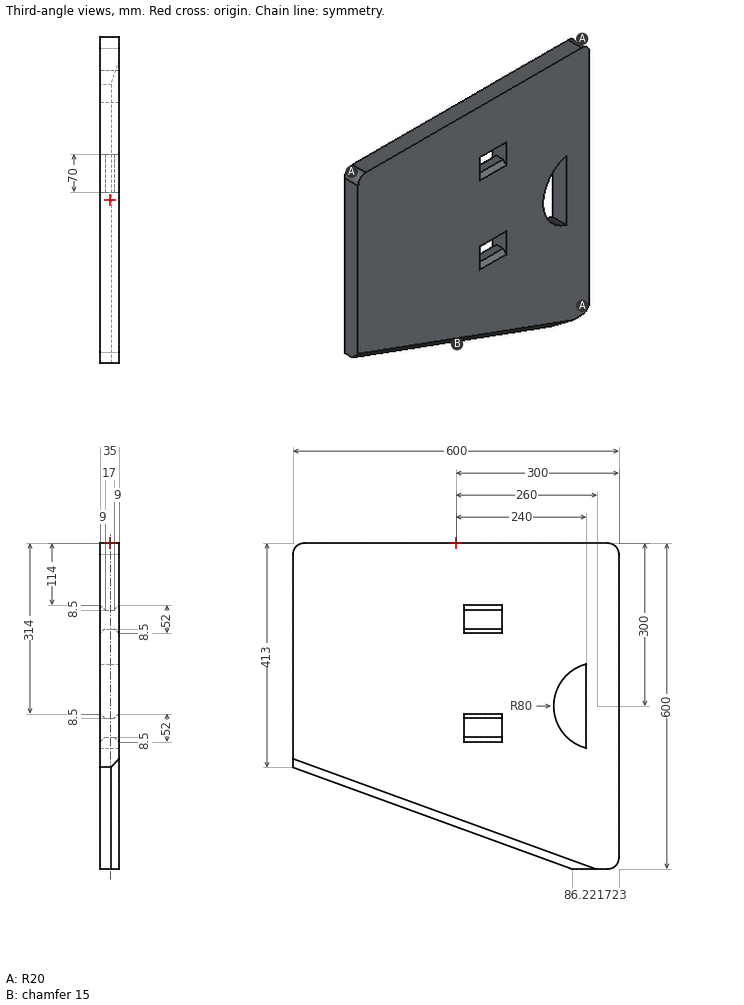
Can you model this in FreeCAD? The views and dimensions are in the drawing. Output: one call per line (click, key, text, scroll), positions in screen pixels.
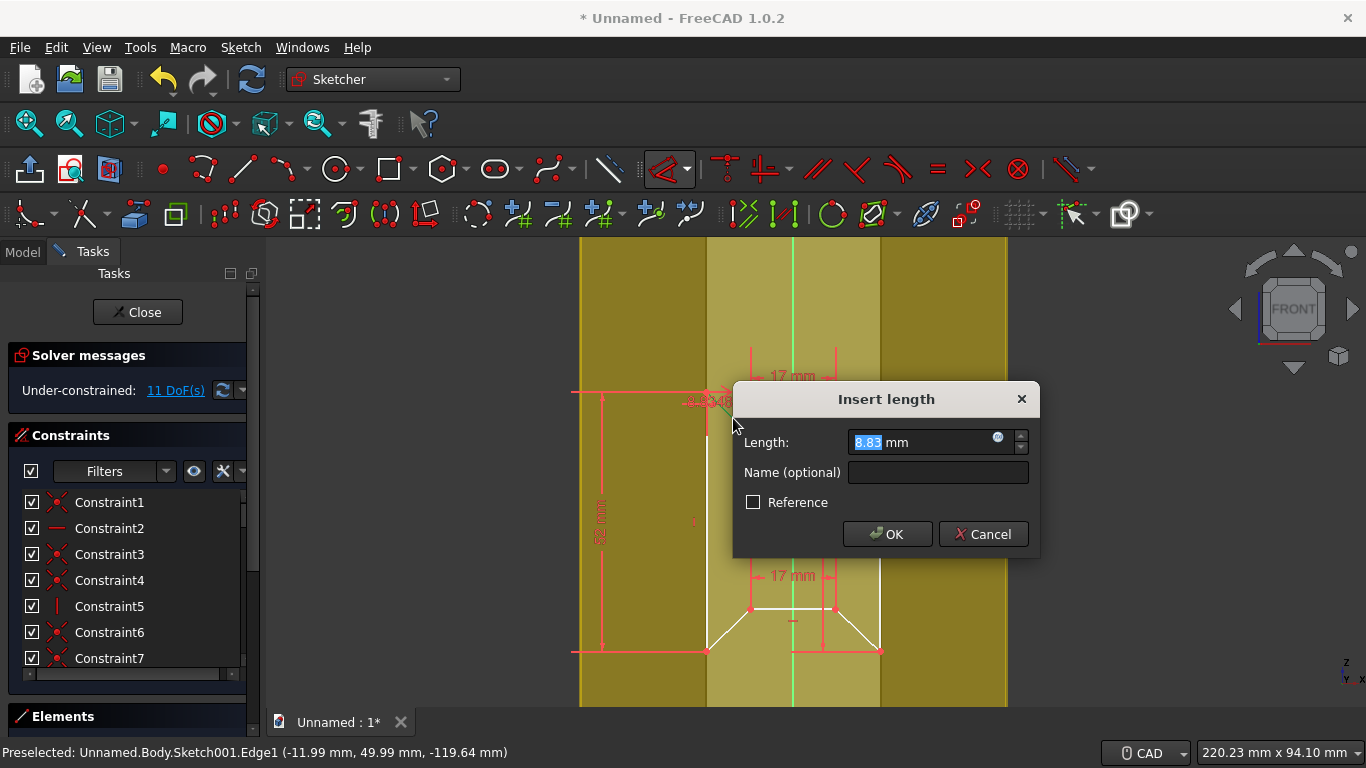
text(9)
key(Return)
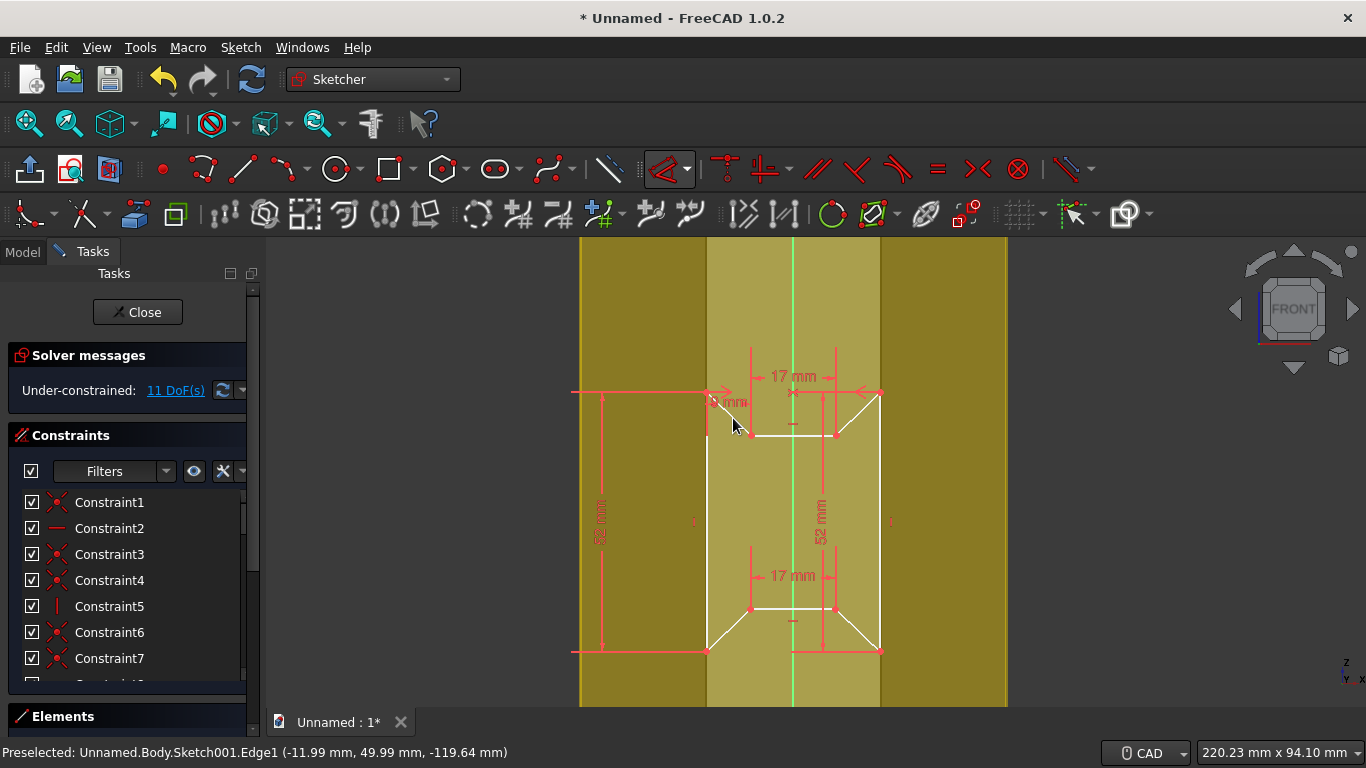
click(849, 422)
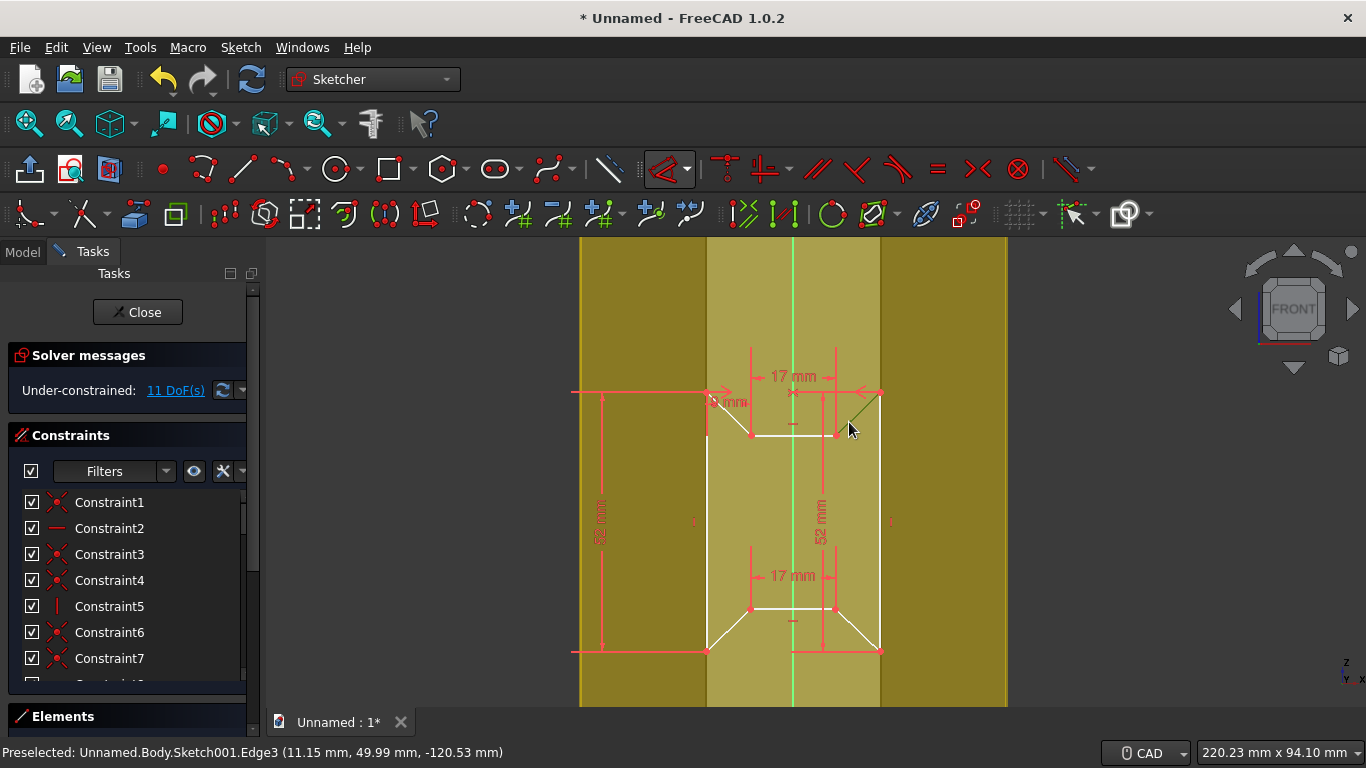
key(l)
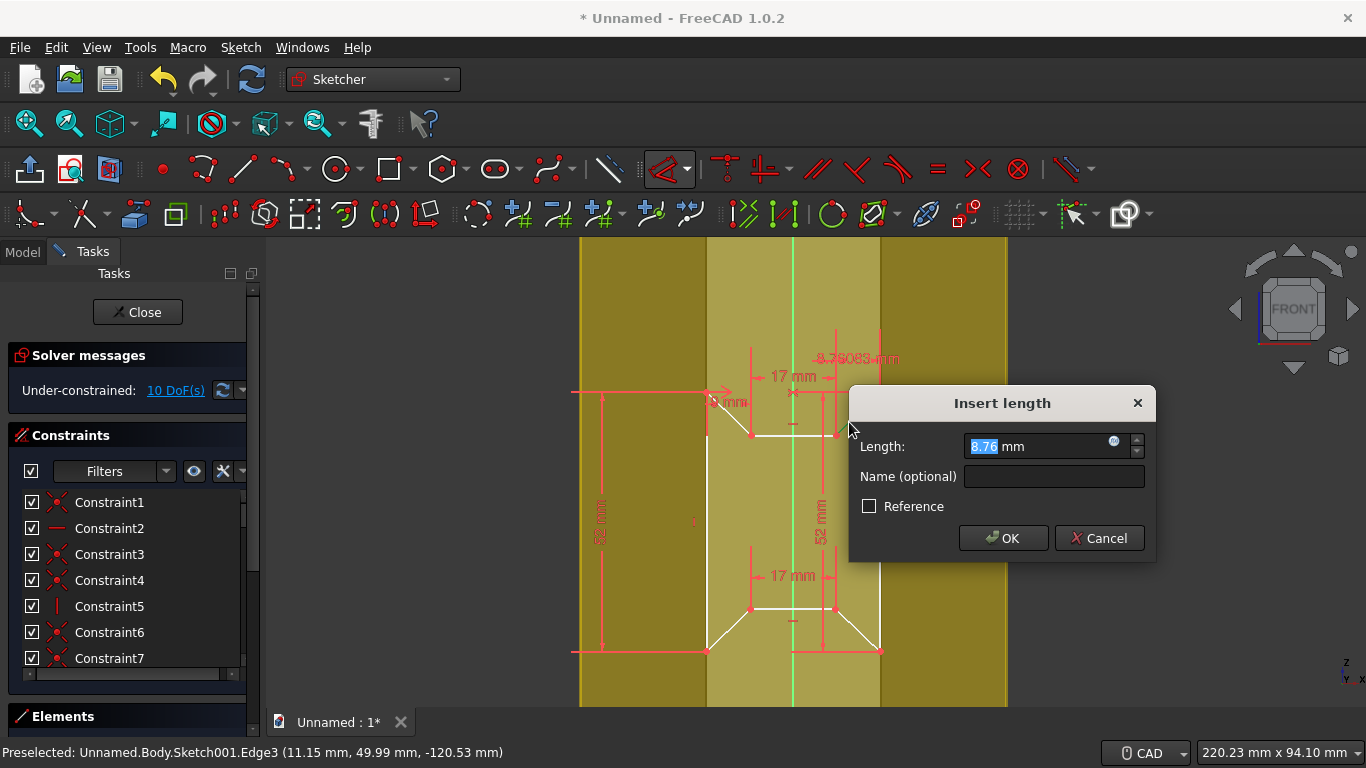
text(9)
key(Return)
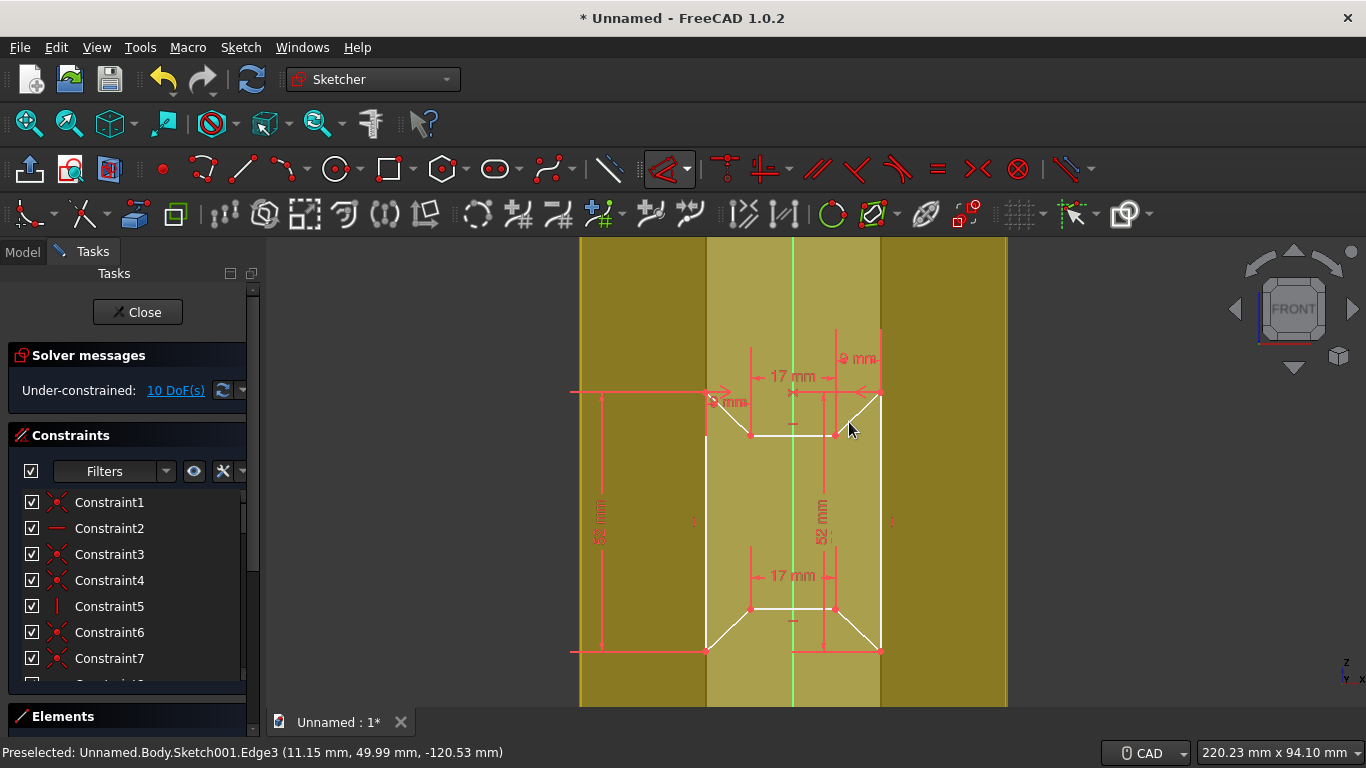
click(867, 639)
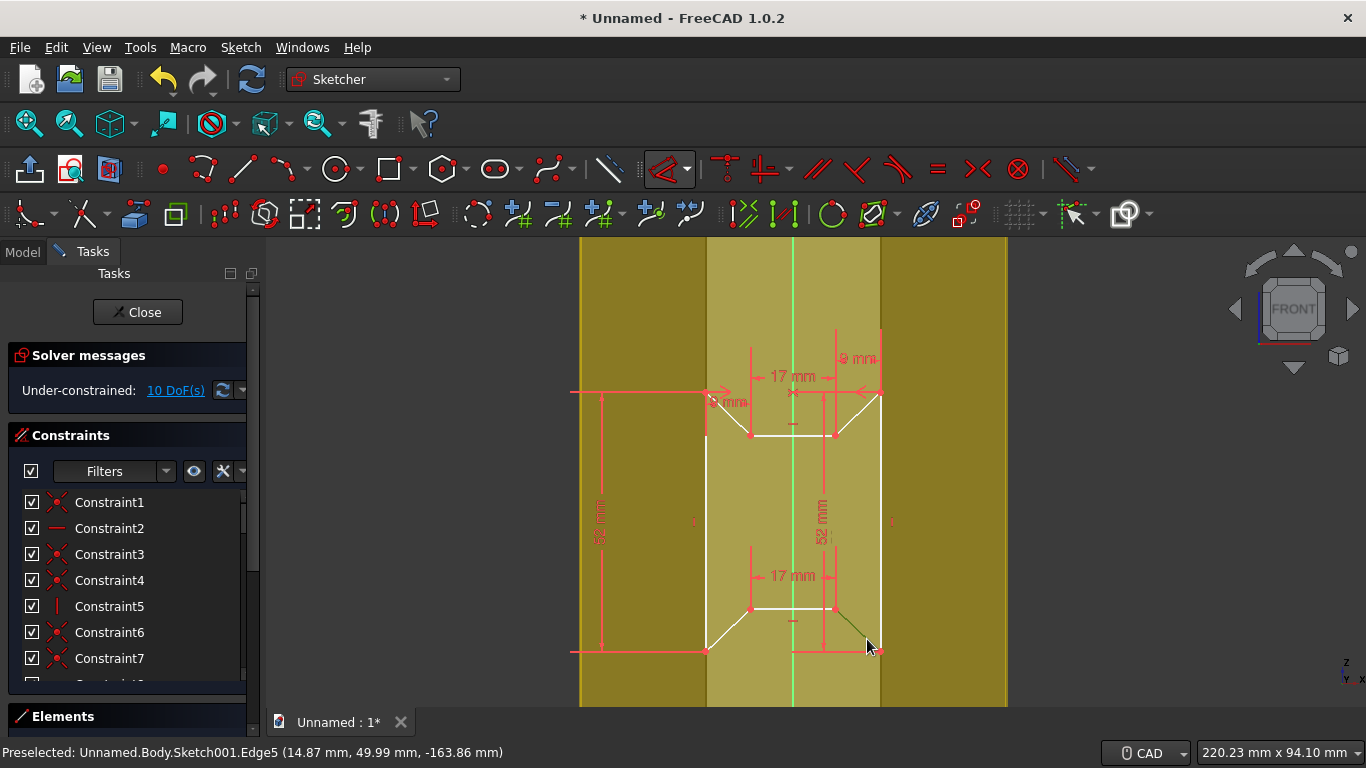
click(690, 170)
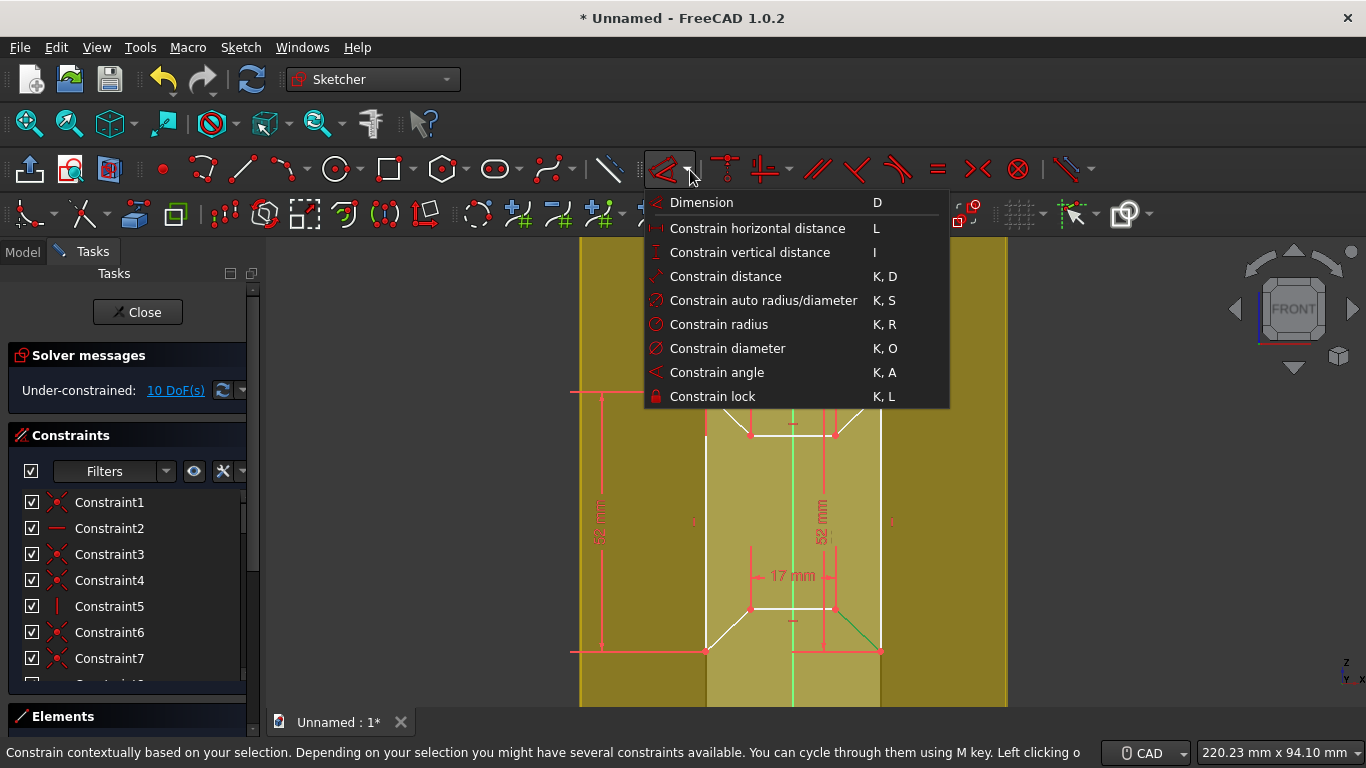
click(797, 228)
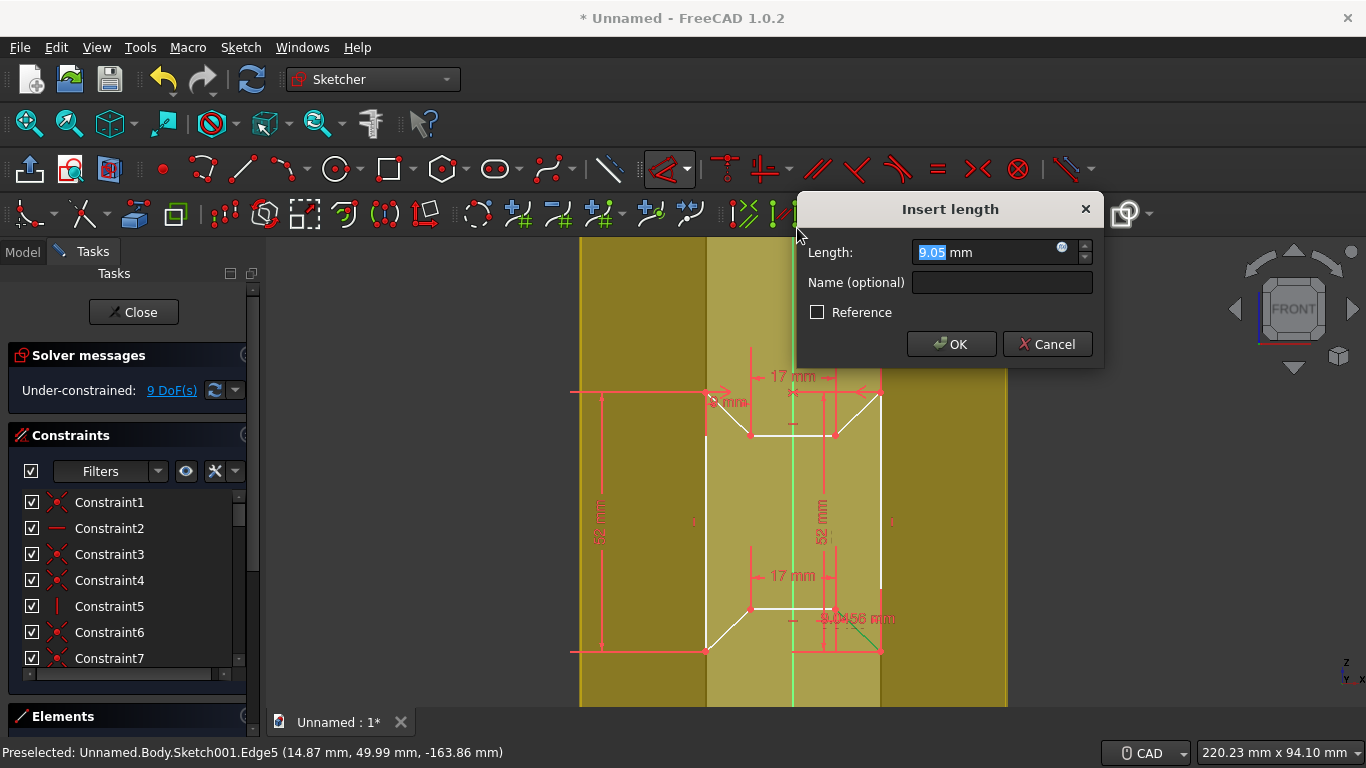
text(9)
key(Return)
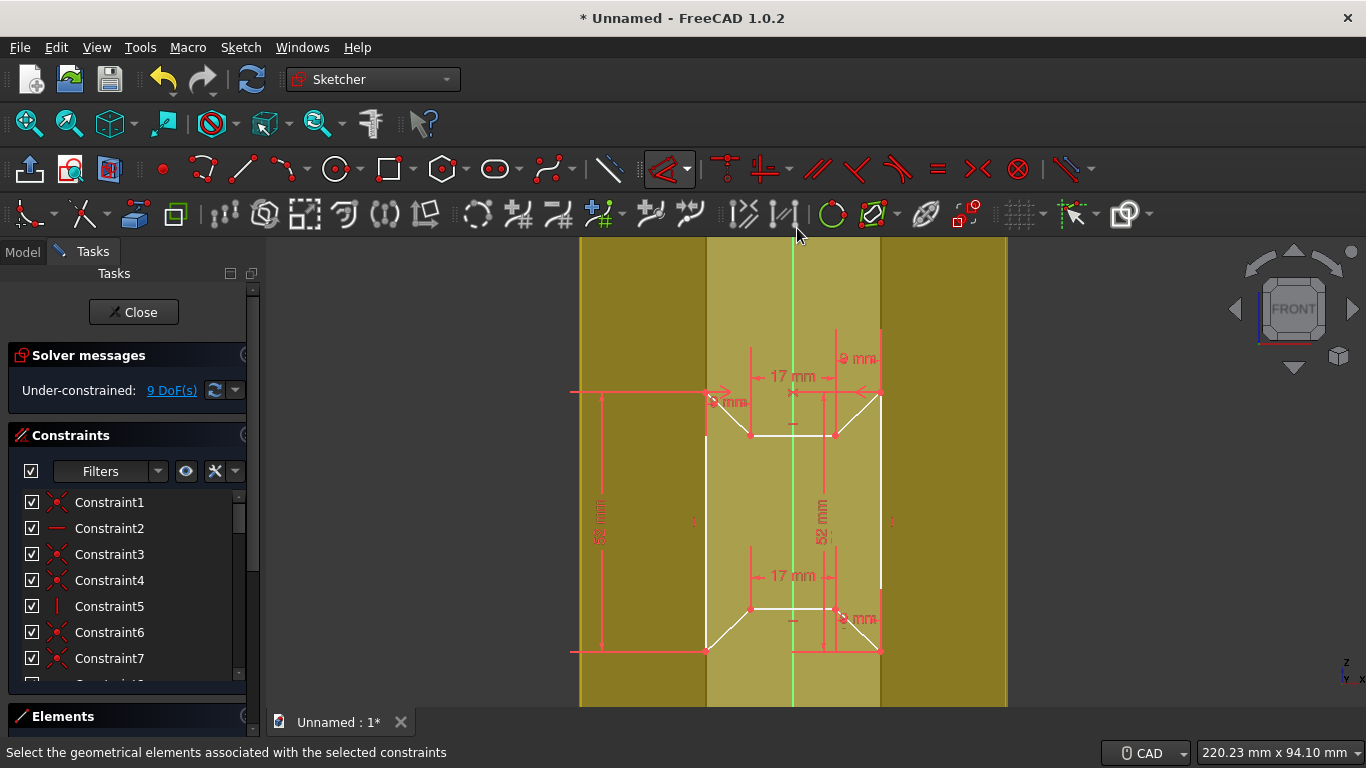
scroll(738, 420, down, 9)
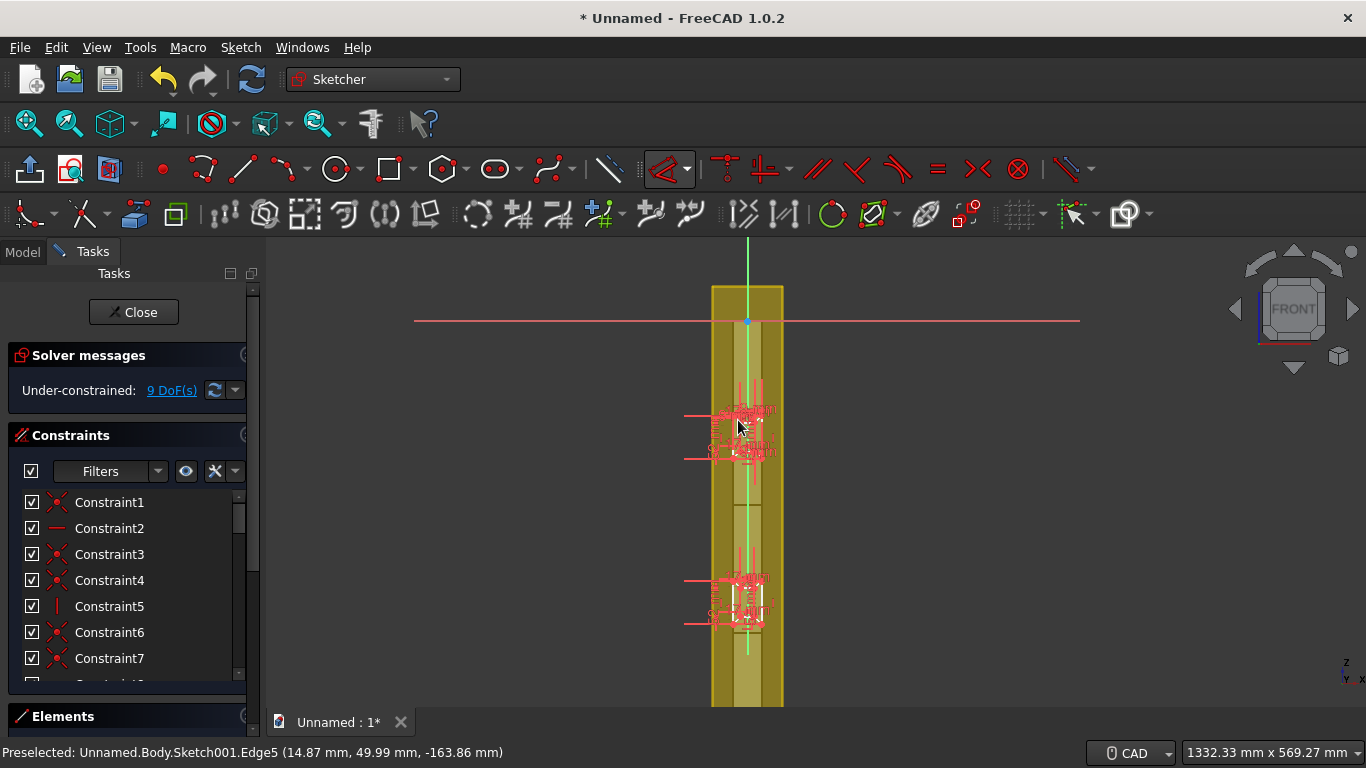
scroll(735, 583, up, 10)